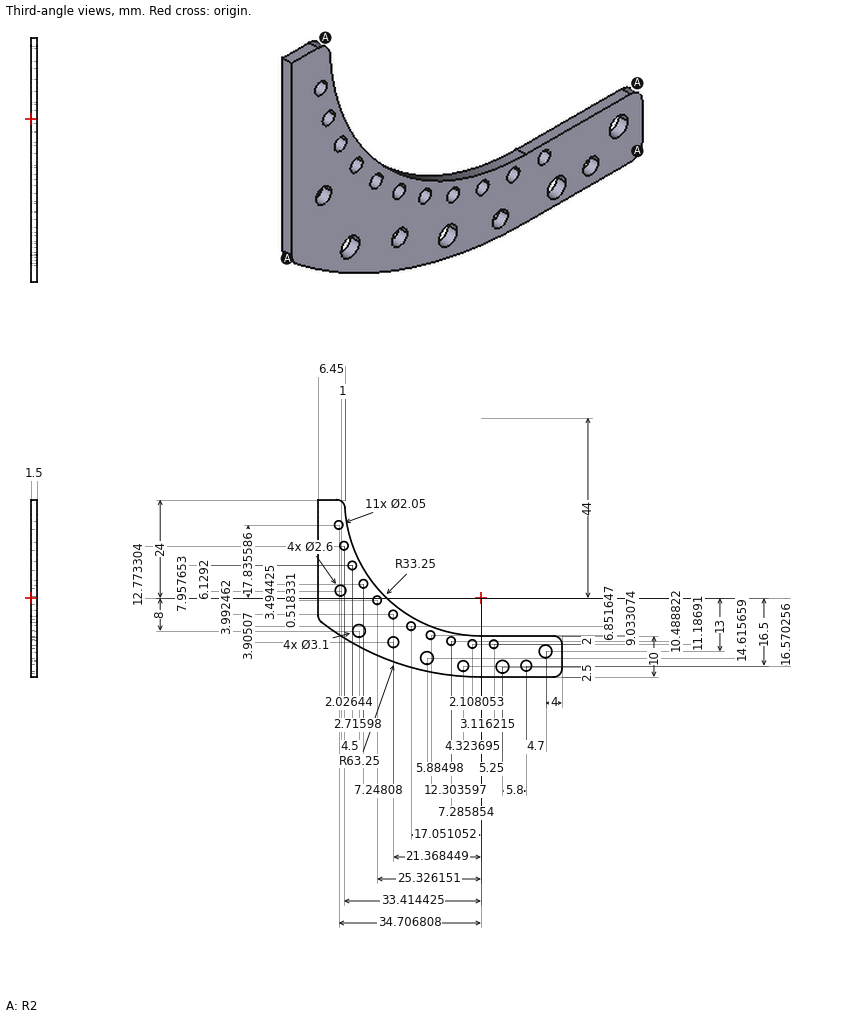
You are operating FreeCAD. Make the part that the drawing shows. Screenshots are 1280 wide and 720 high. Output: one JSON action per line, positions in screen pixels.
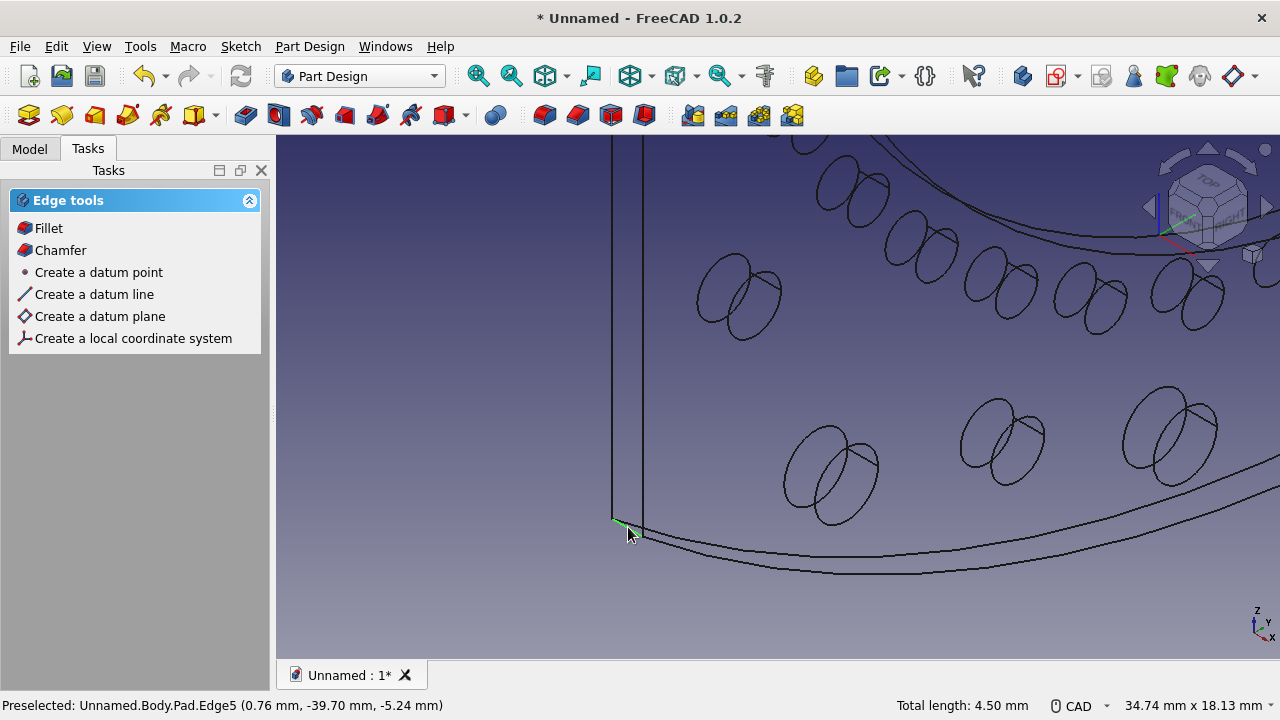
{"action": "left_click", "coordinate": [479, 76]}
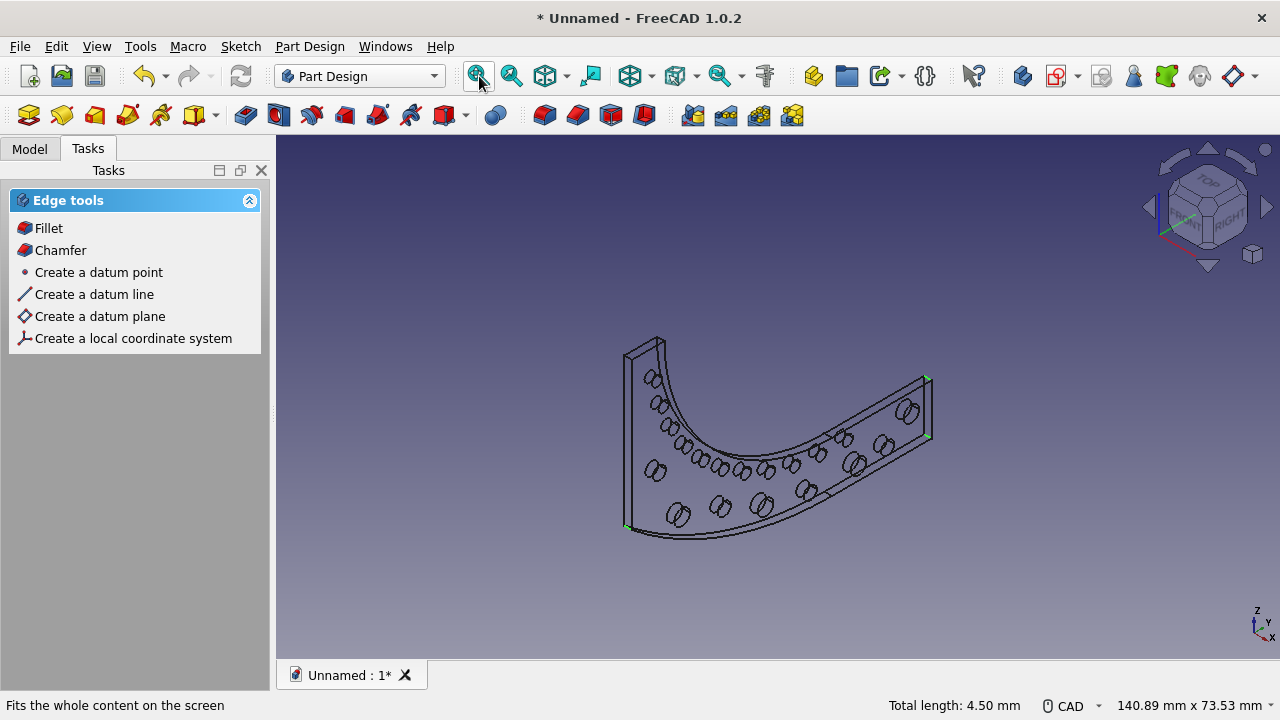
{"action": "key", "text": "2"}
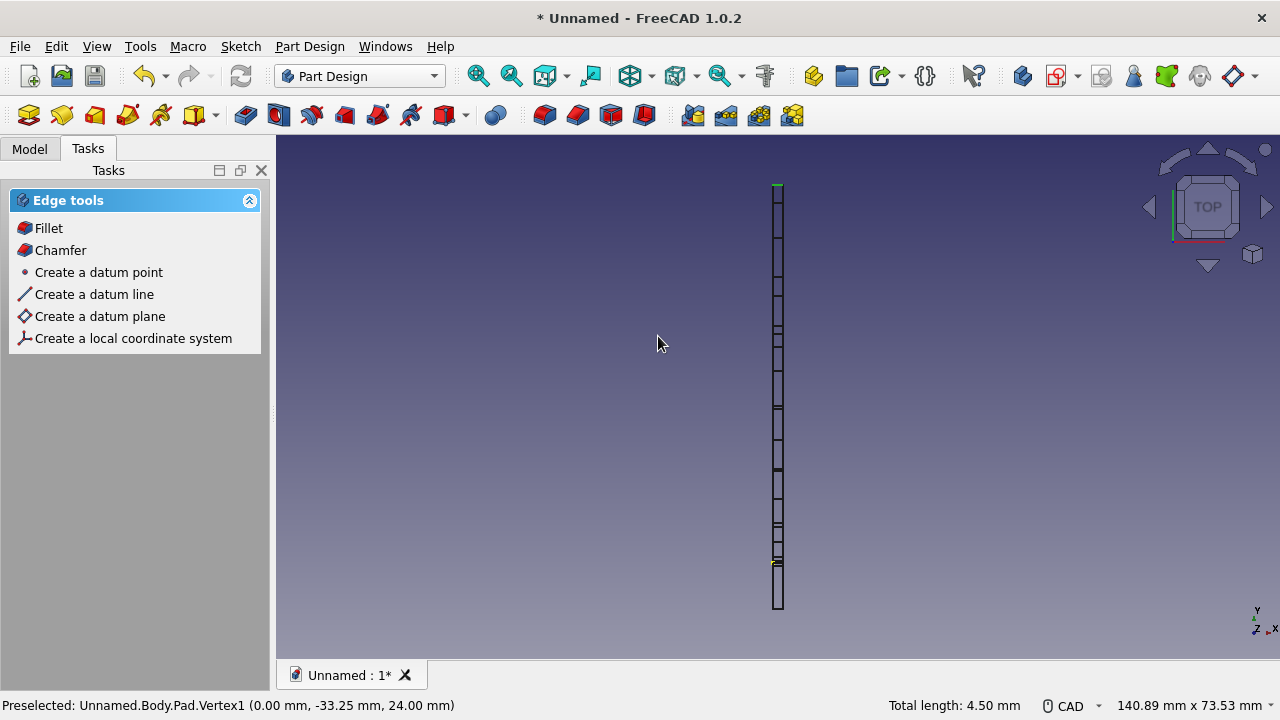
{"action": "left_click", "coordinate": [778, 562], "text": "ctrl"}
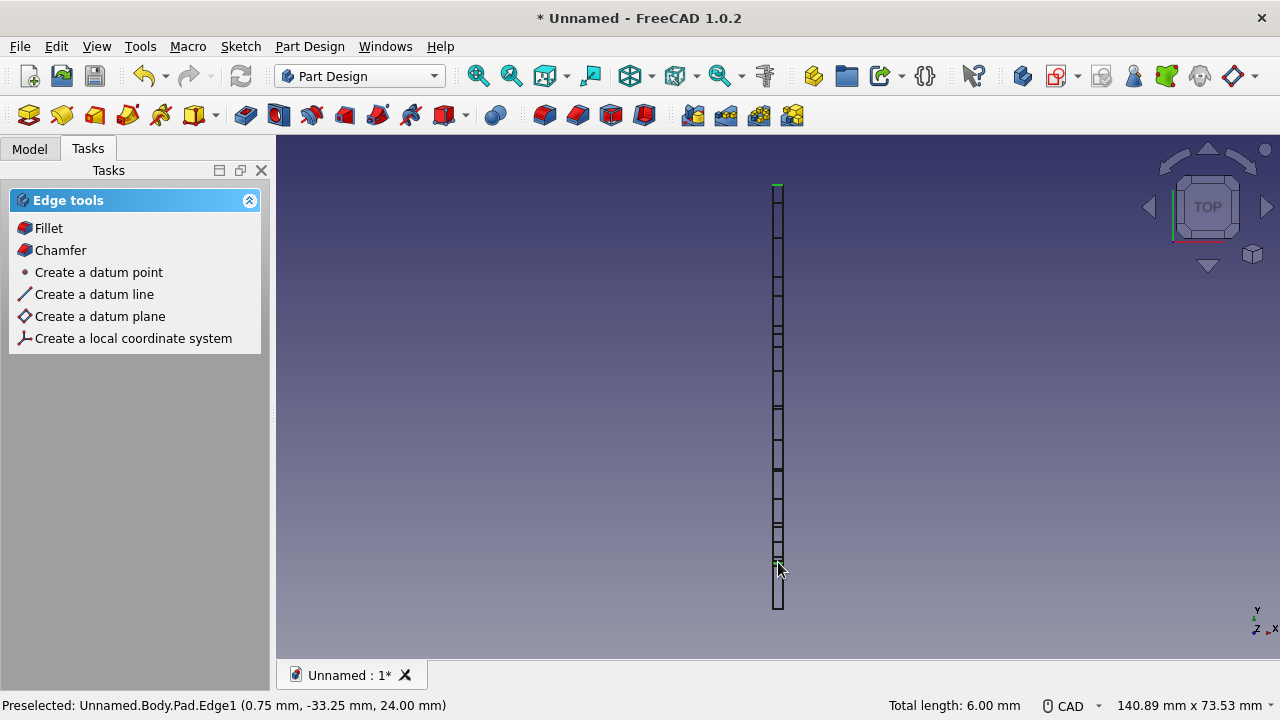
{"action": "key", "text": "v 1"}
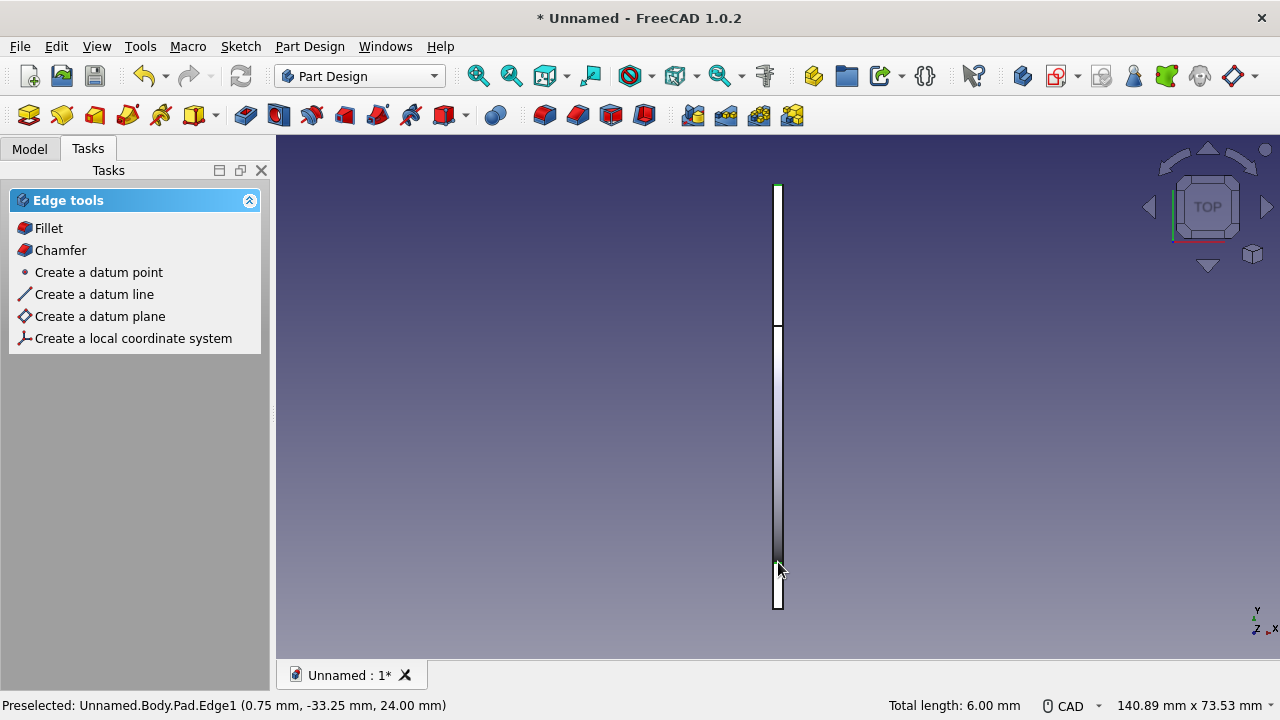
{"action": "left_click", "coordinate": [545, 116]}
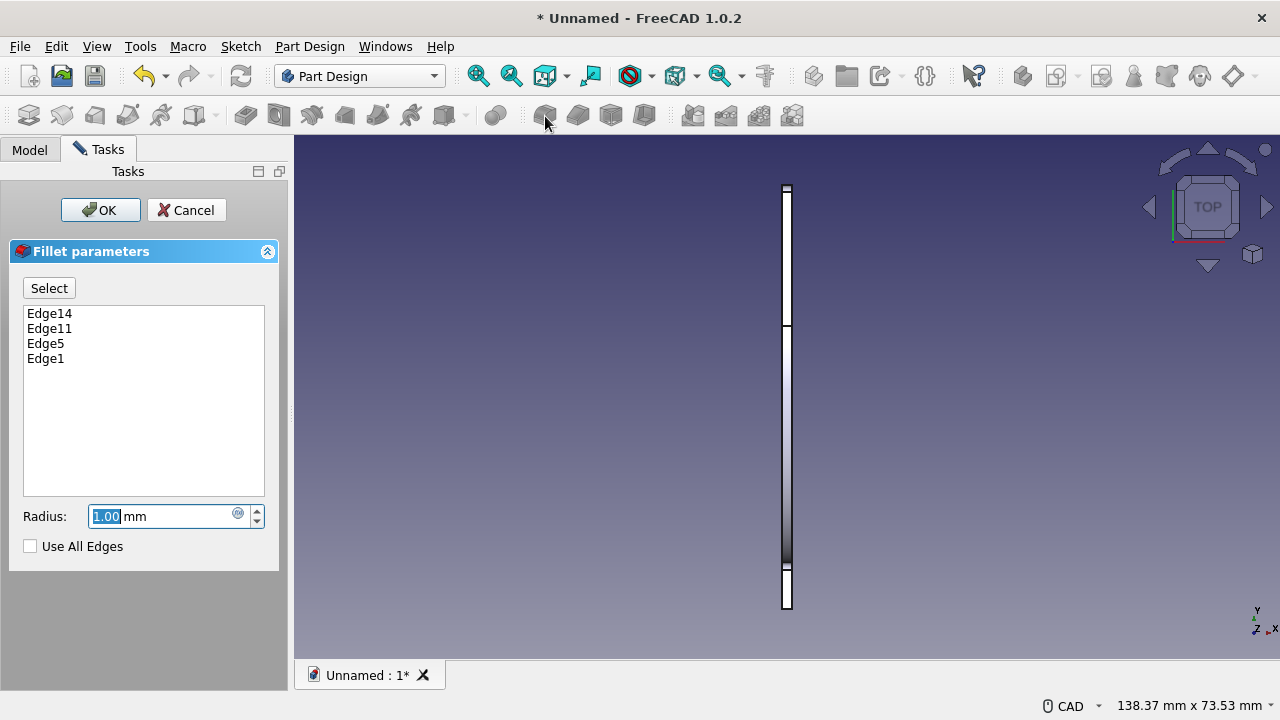
{"action": "type", "text": "2"}
{"action": "key", "text": "Tab"}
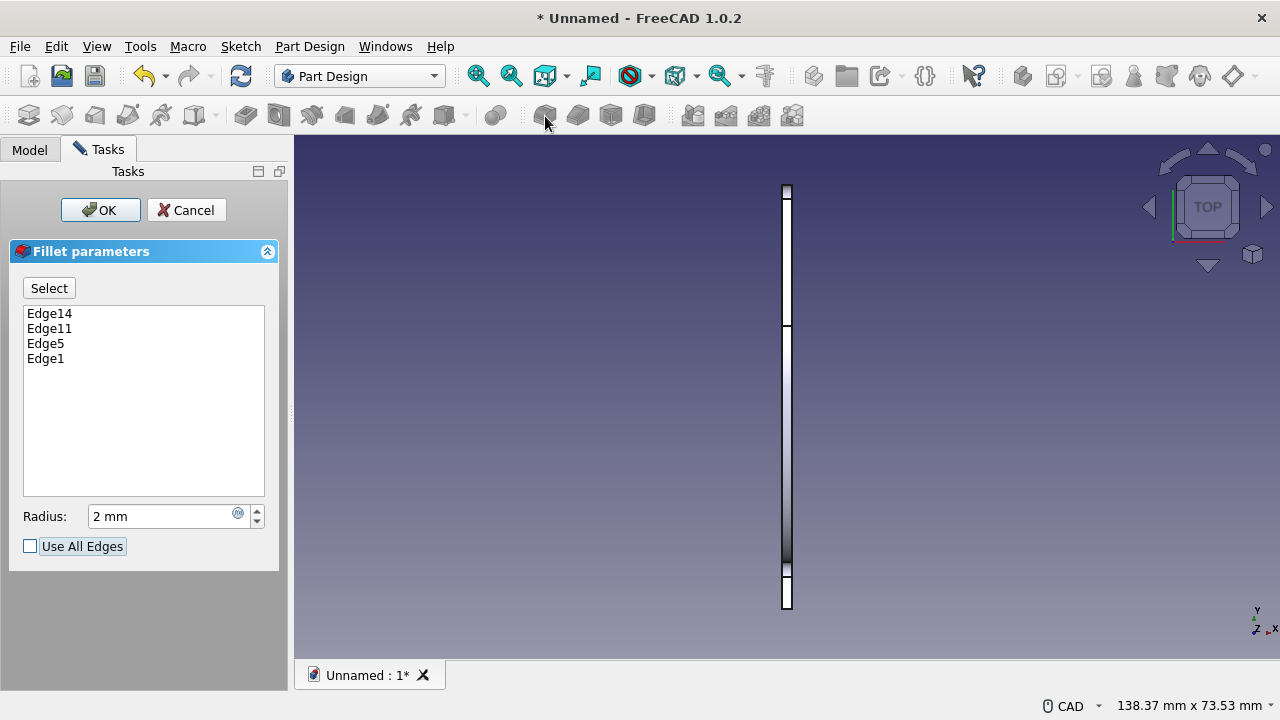
{"action": "left_click", "coordinate": [101, 210]}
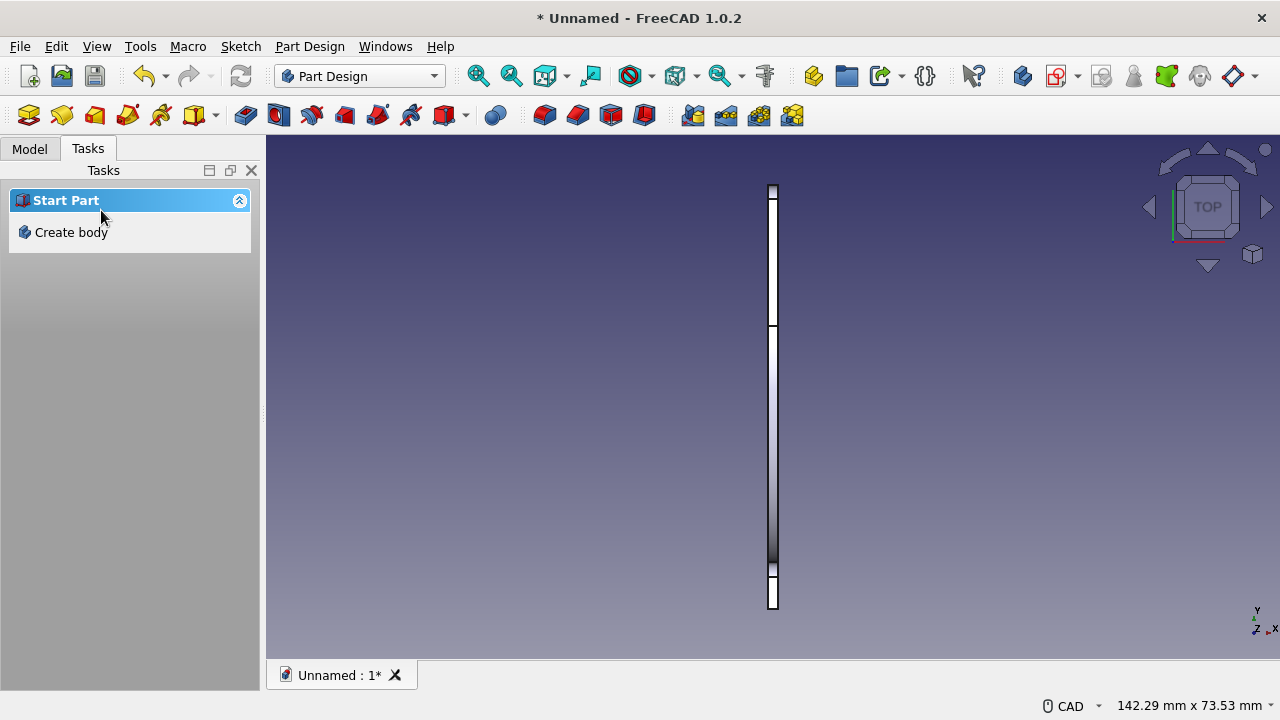
{"action": "key", "text": "0"}